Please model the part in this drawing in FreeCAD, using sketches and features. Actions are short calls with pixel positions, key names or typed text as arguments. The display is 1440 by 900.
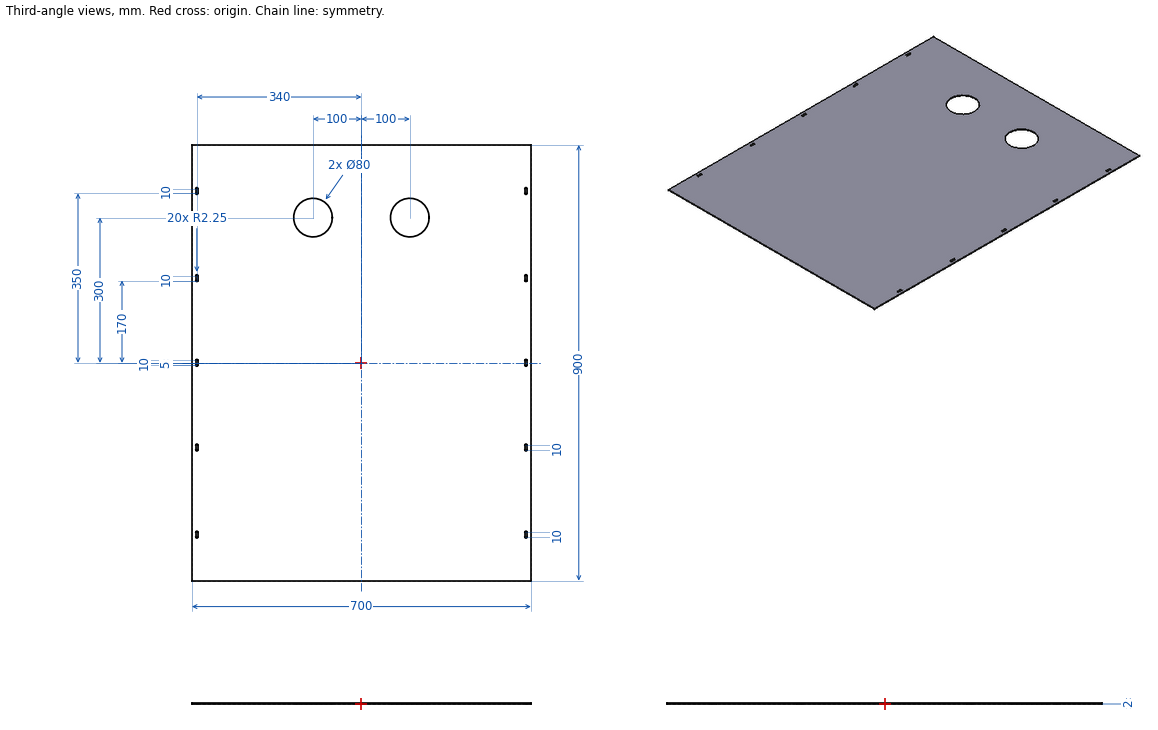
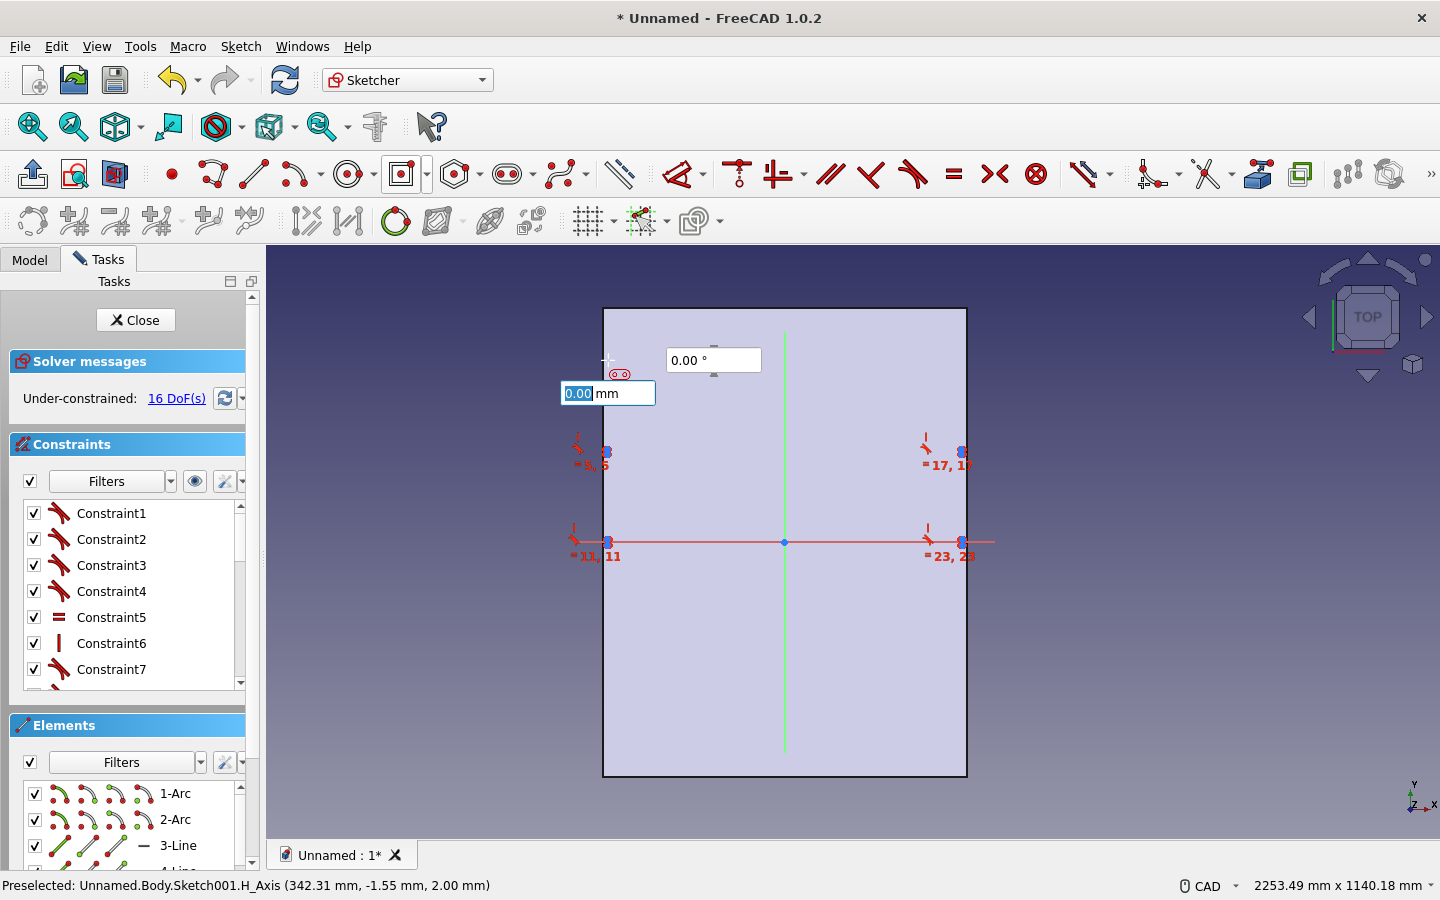
scroll(608, 355, up, 6)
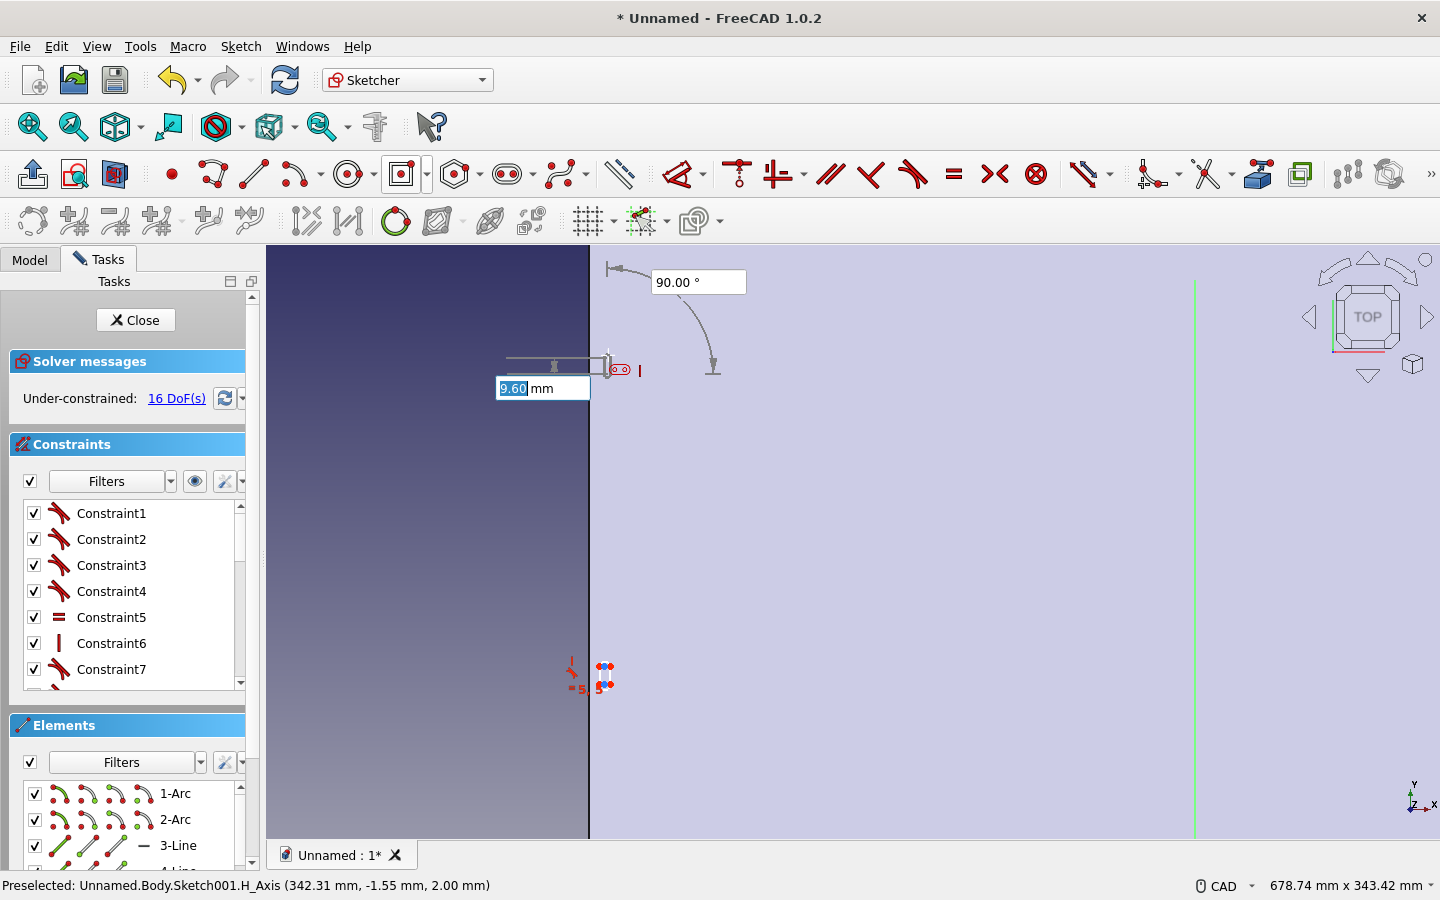
click(607, 354)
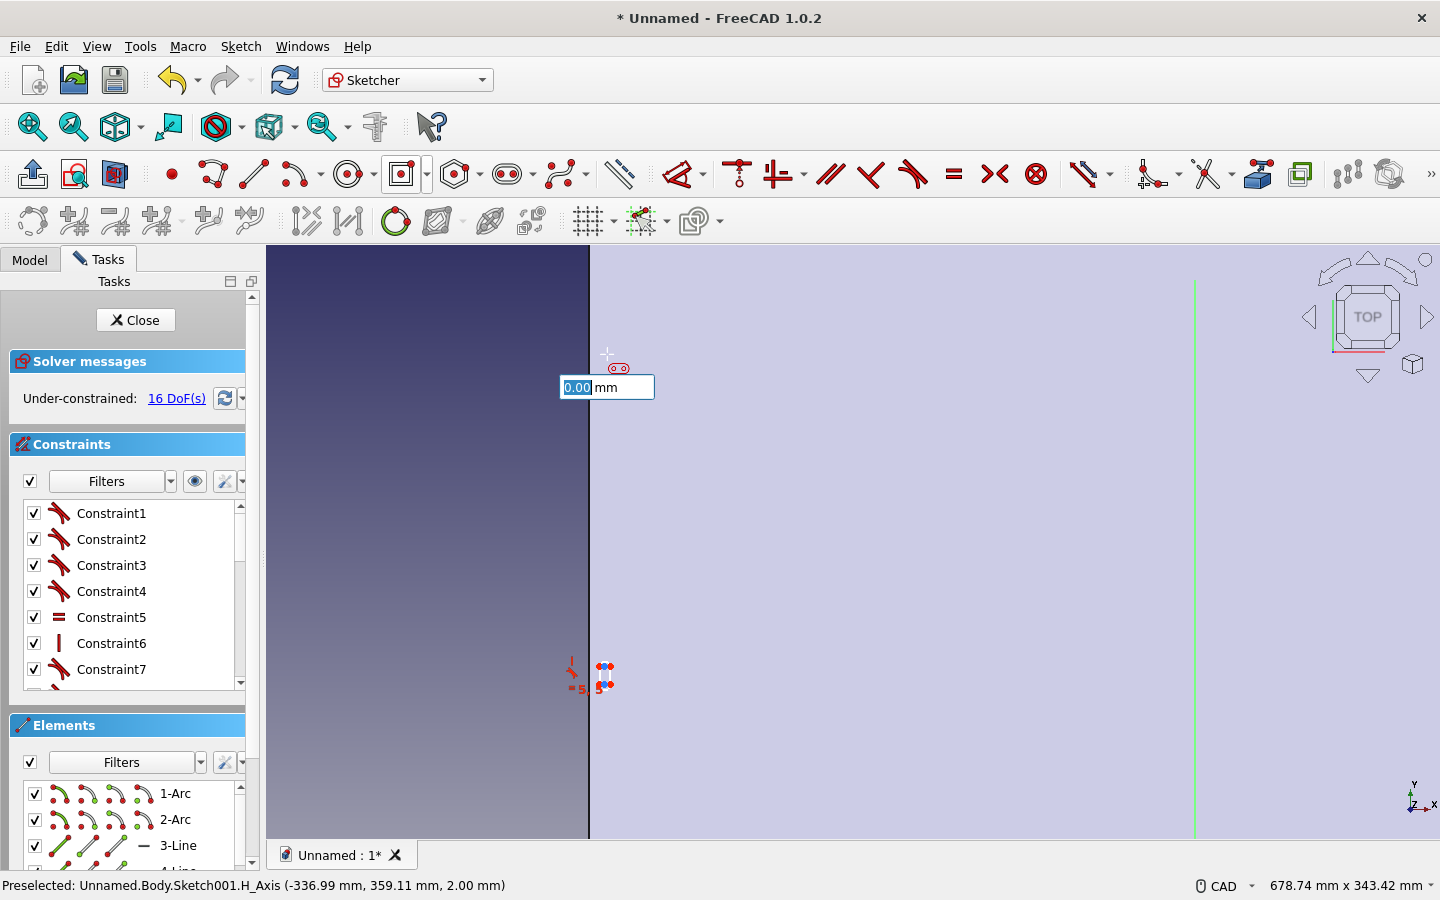
scroll(603, 363, up, 8)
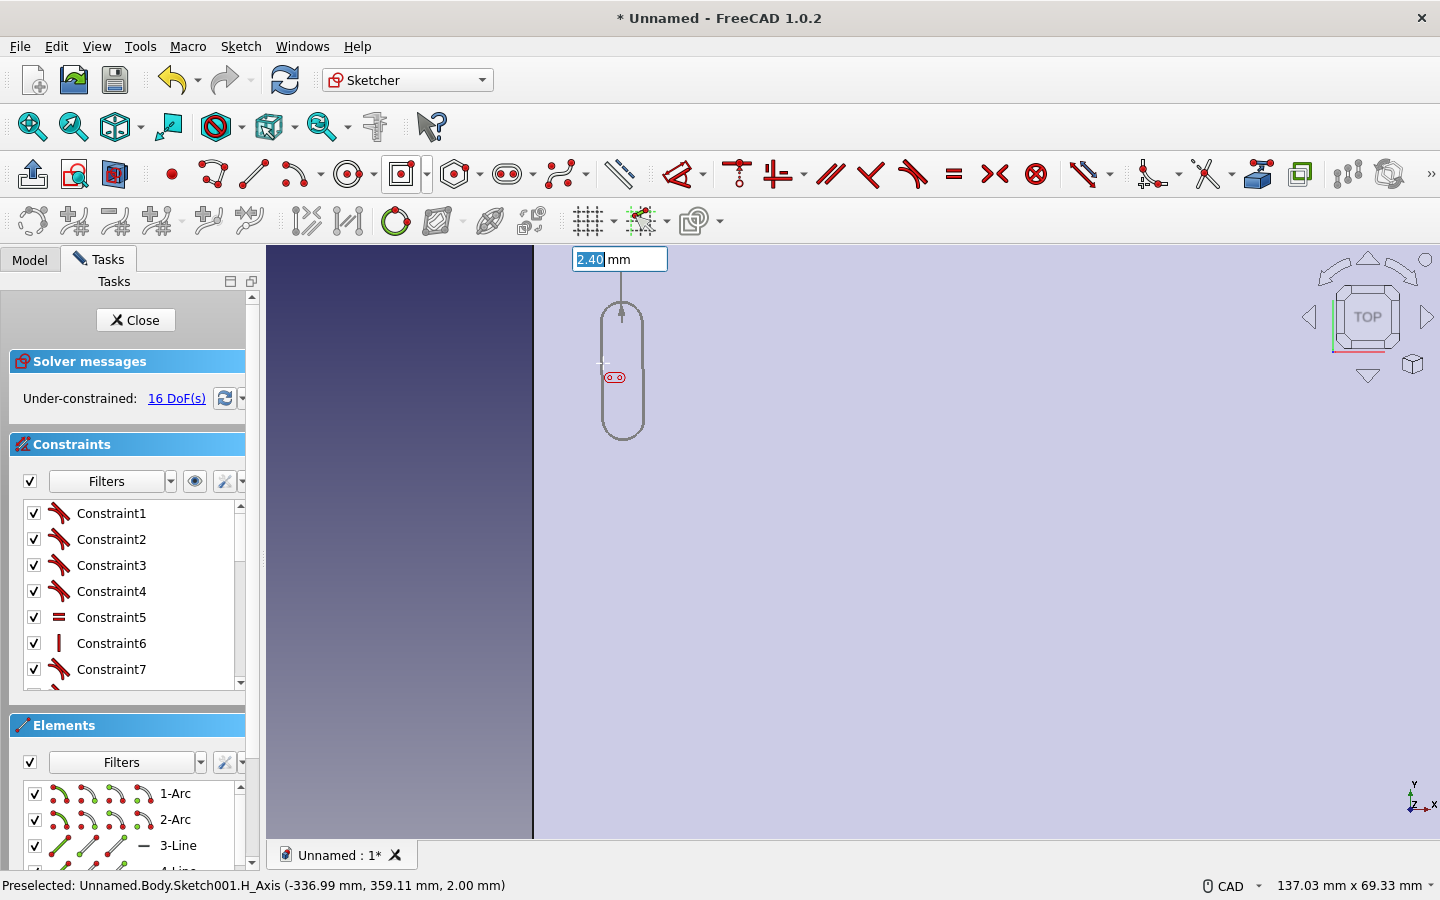
click(600, 362)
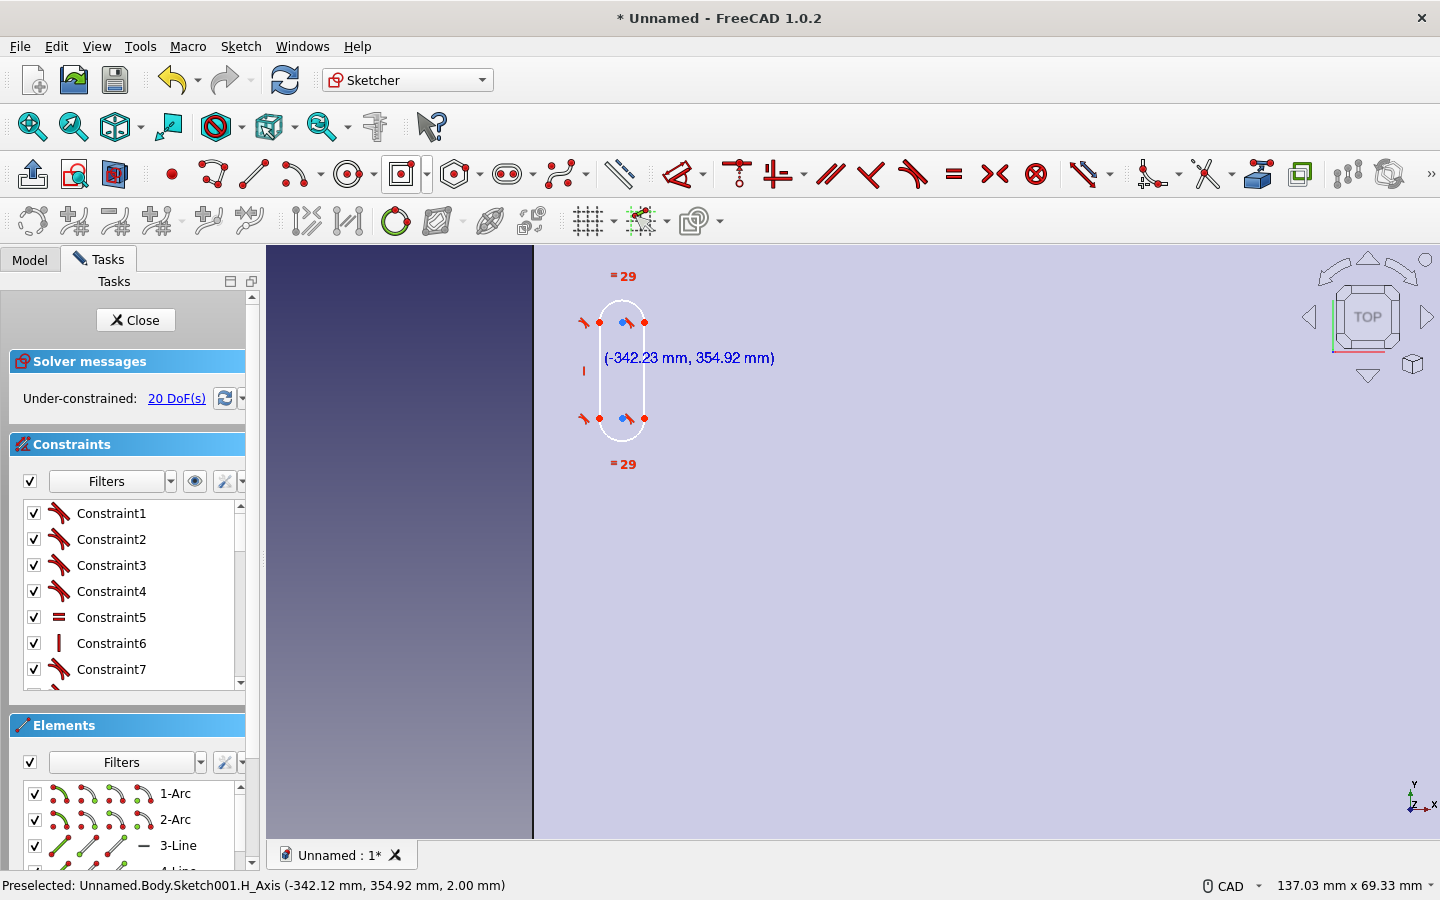
scroll(607, 357, down, 14)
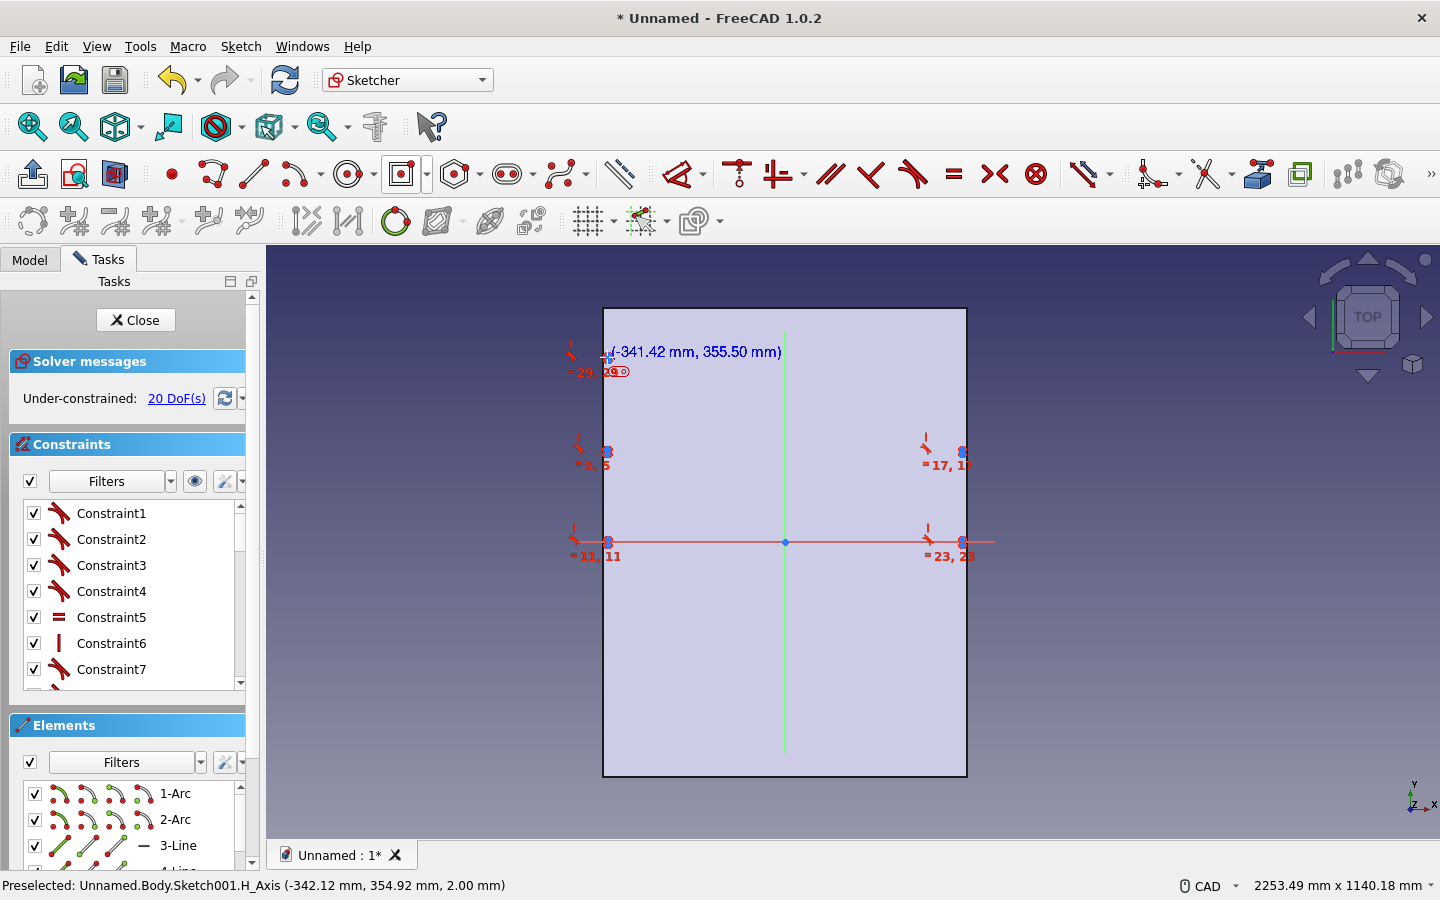
scroll(962, 636, up, 15)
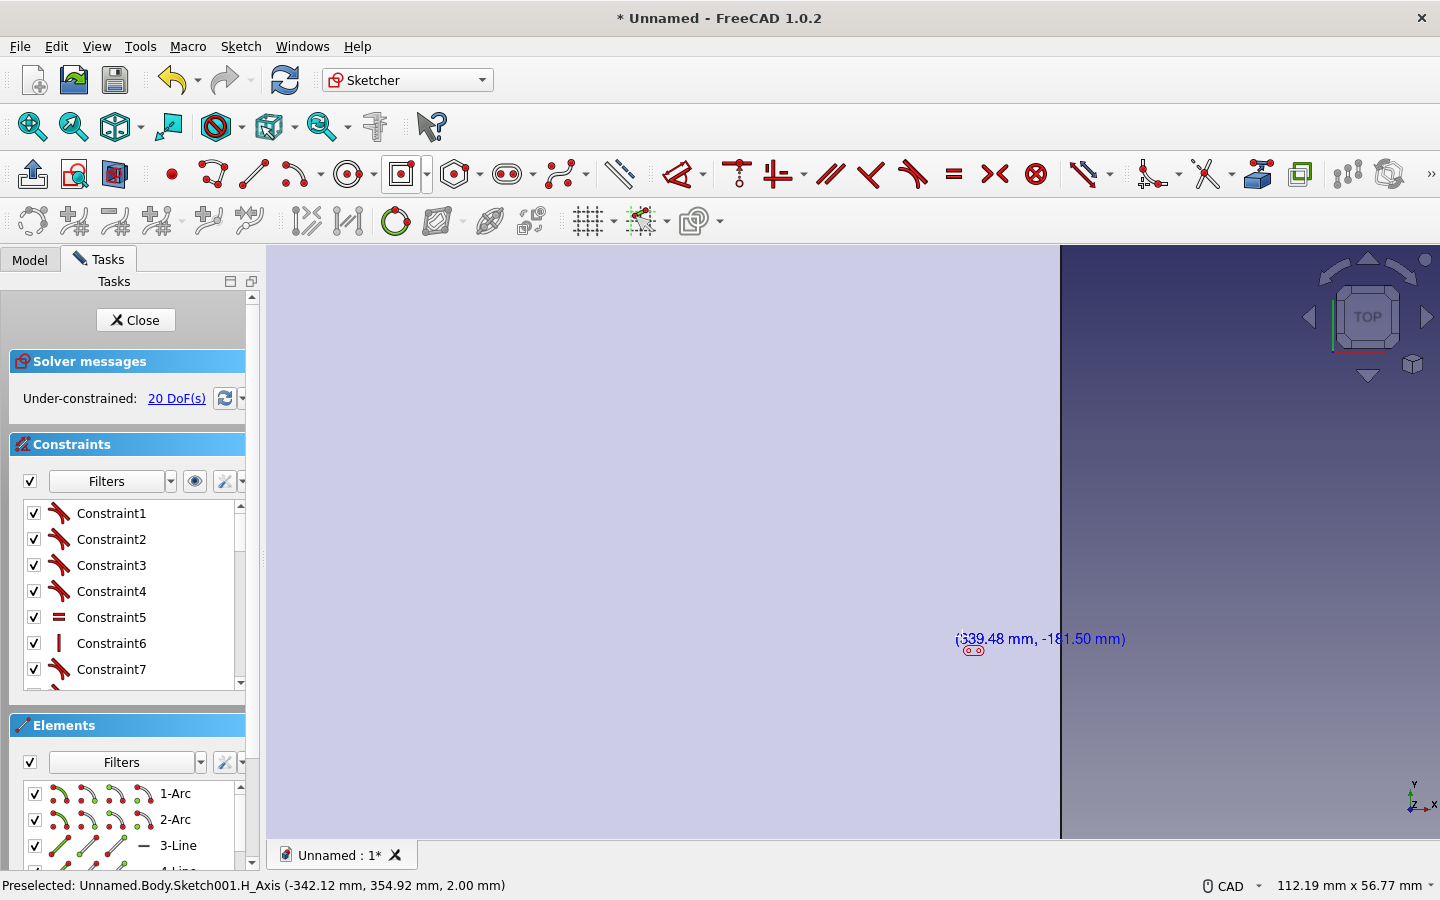
scroll(962, 636, down, 15)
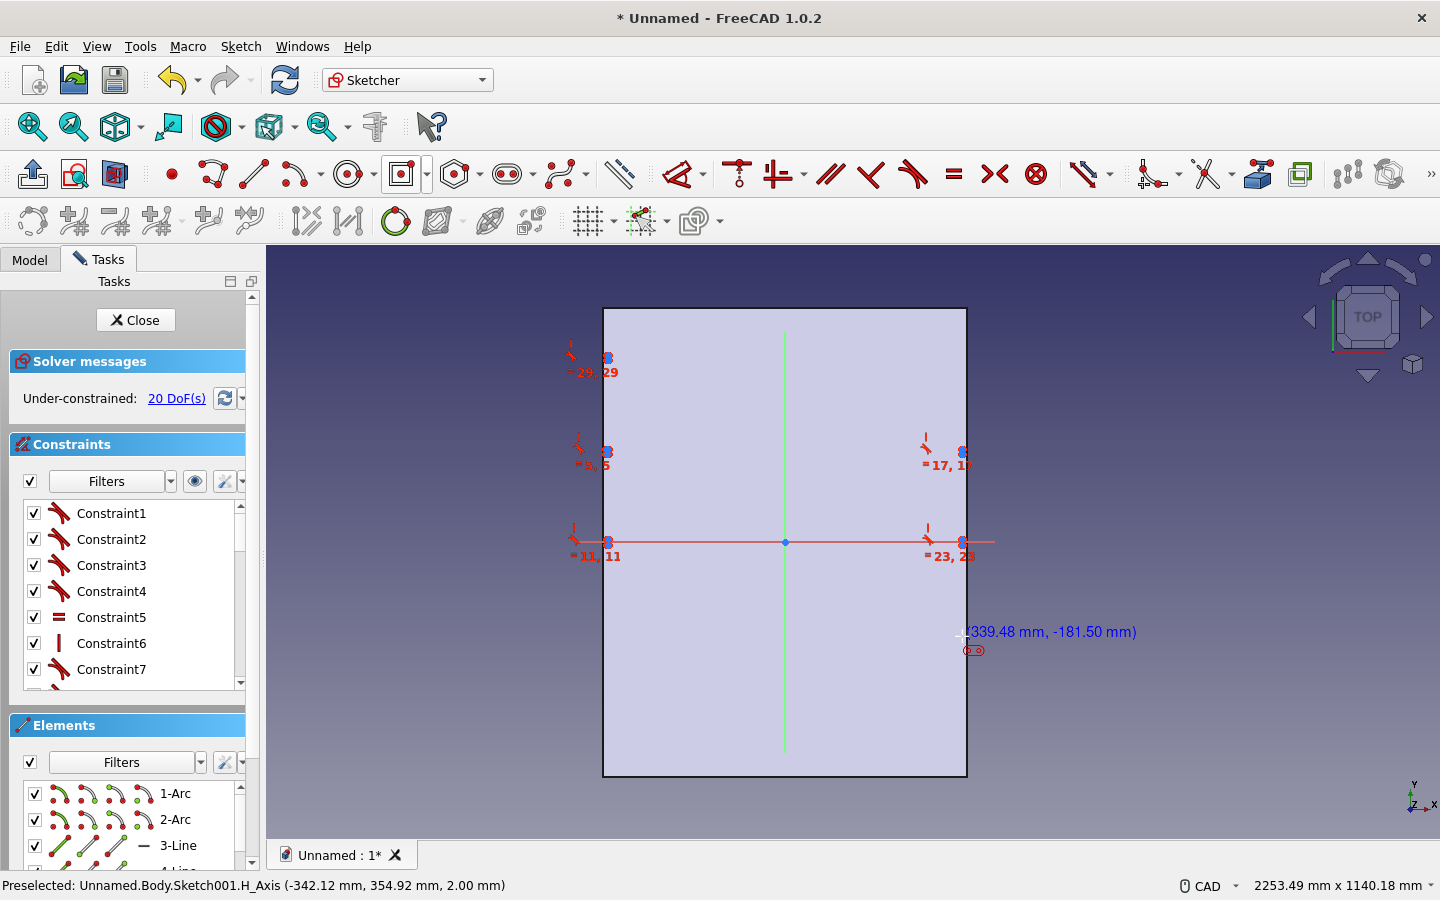
click(962, 636)